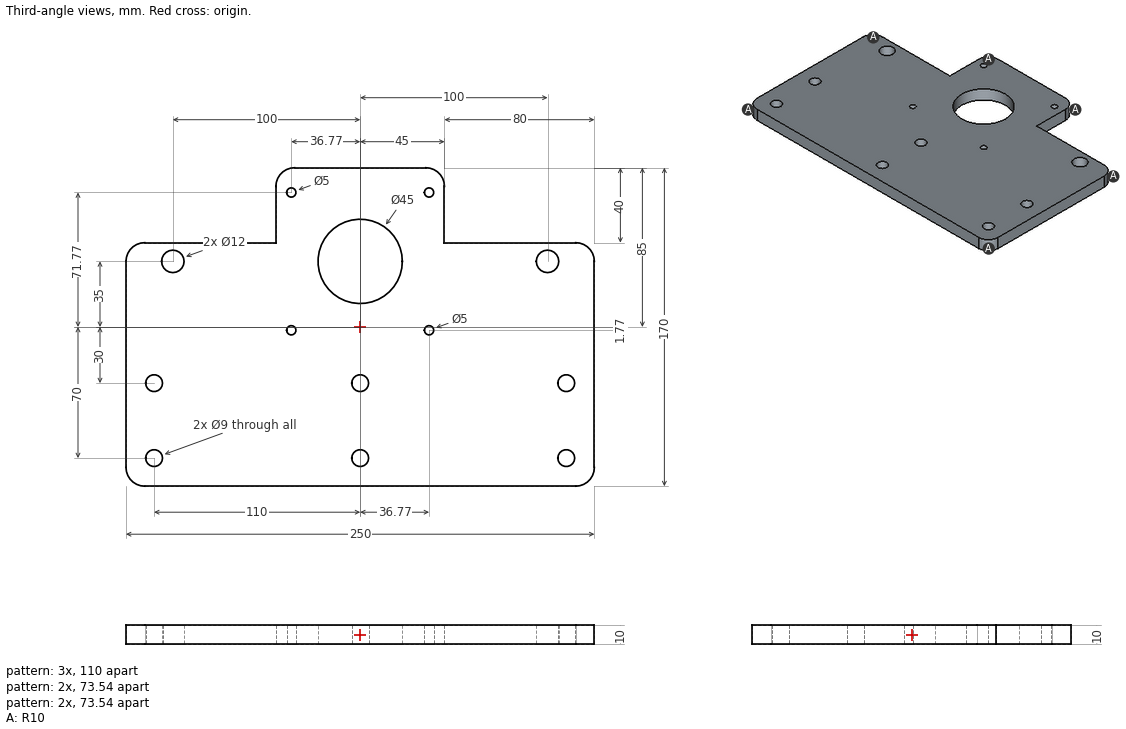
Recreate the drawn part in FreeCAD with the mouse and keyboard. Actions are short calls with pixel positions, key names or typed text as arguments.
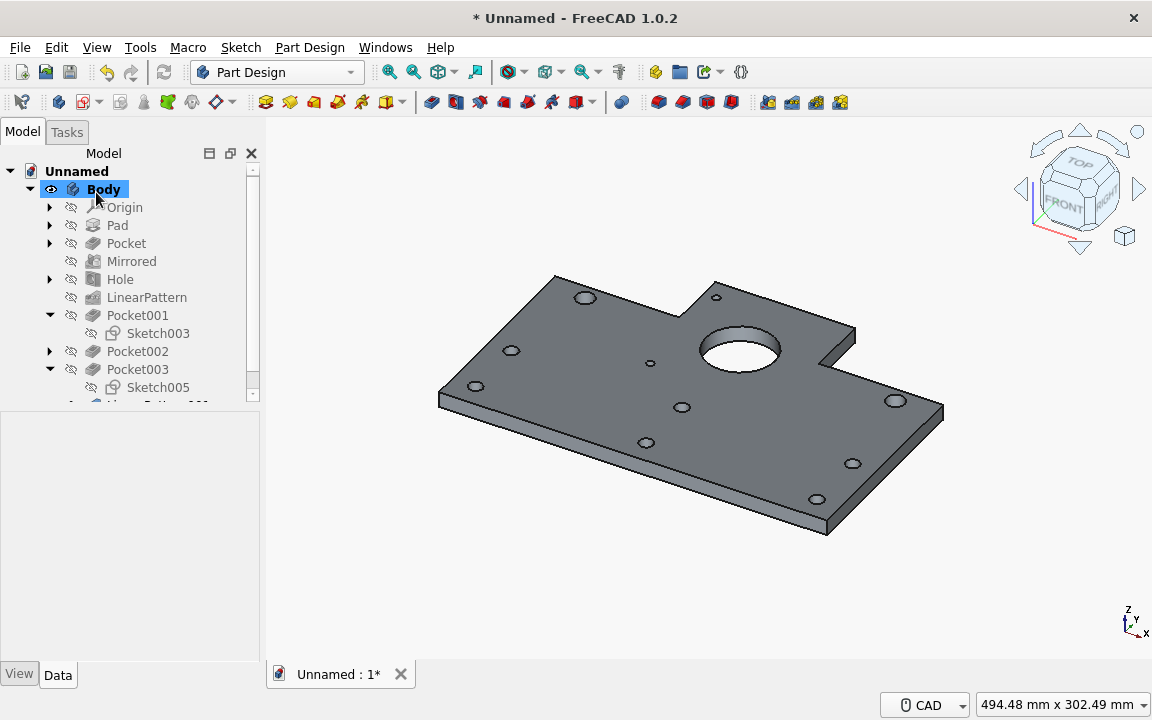
click(116, 369)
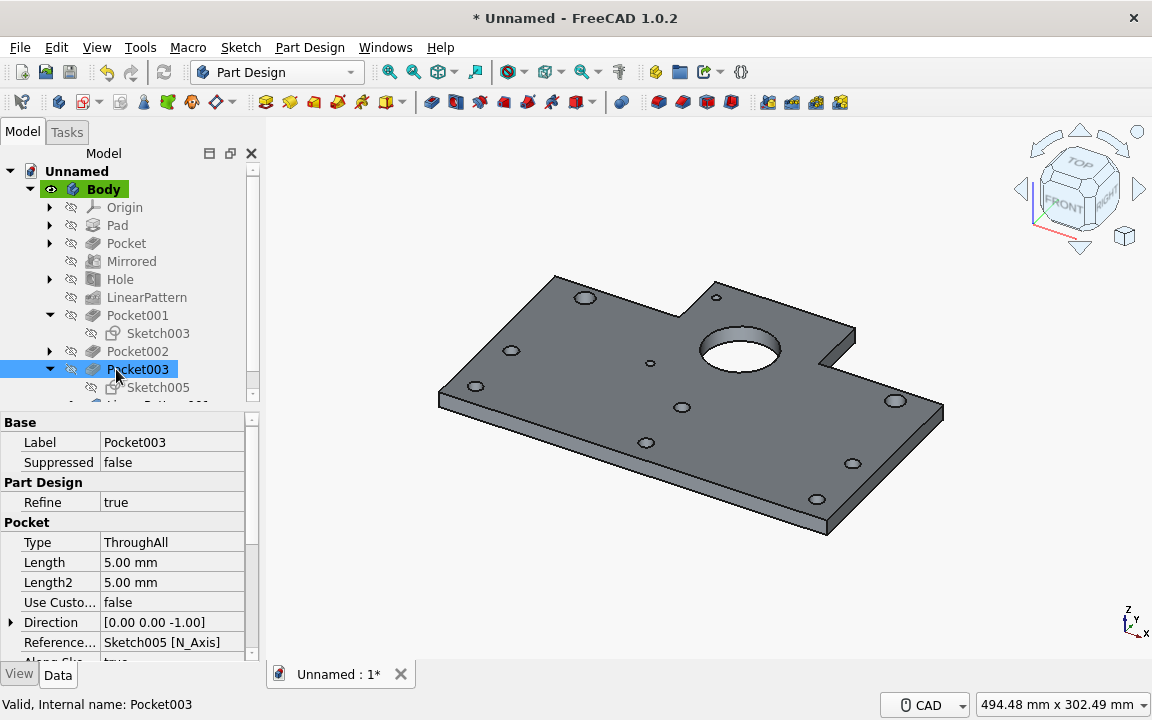
click(792, 102)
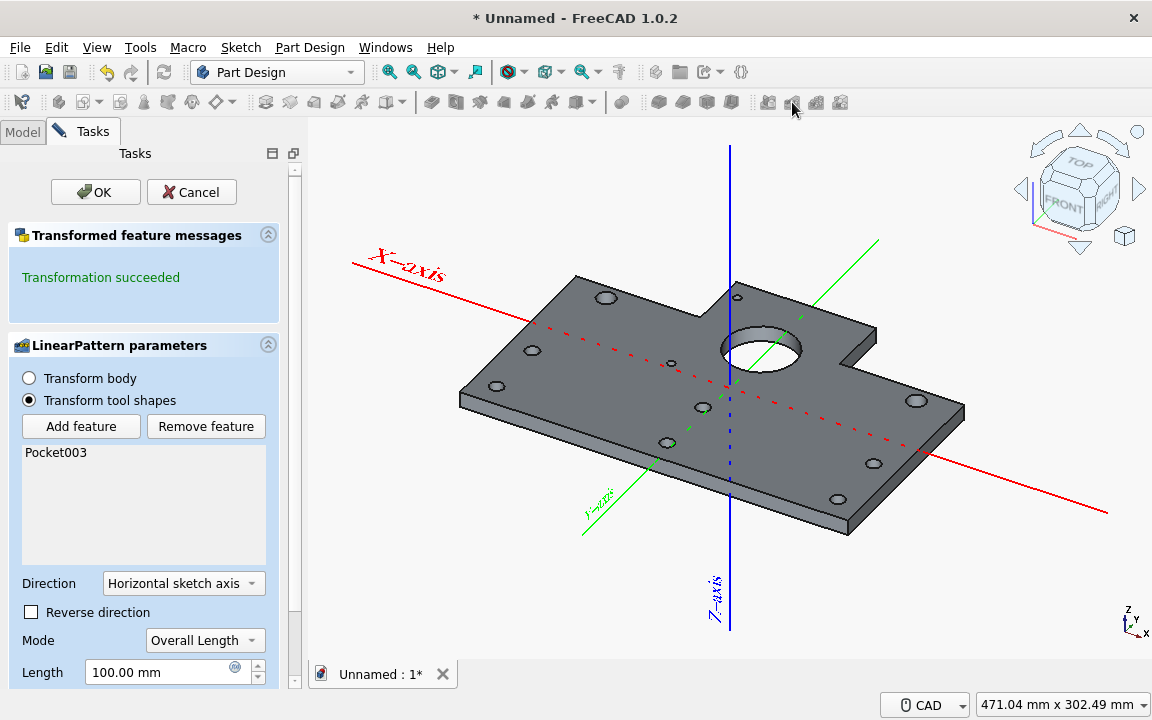
click(184, 584)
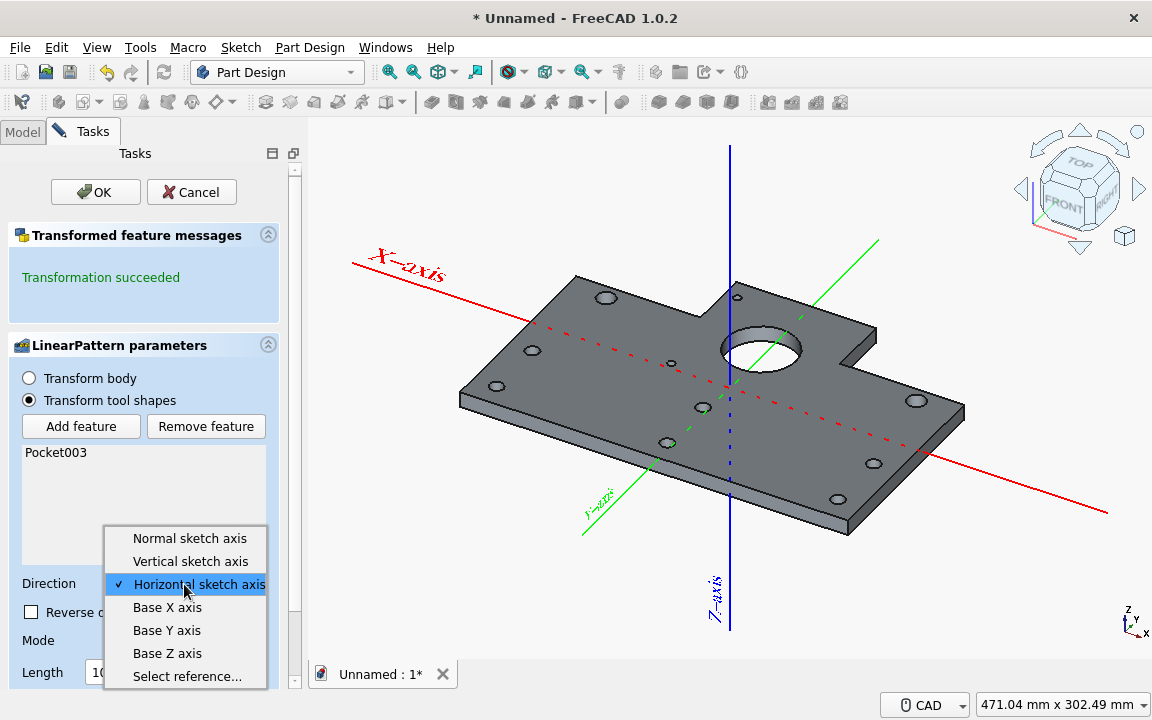
click(184, 608)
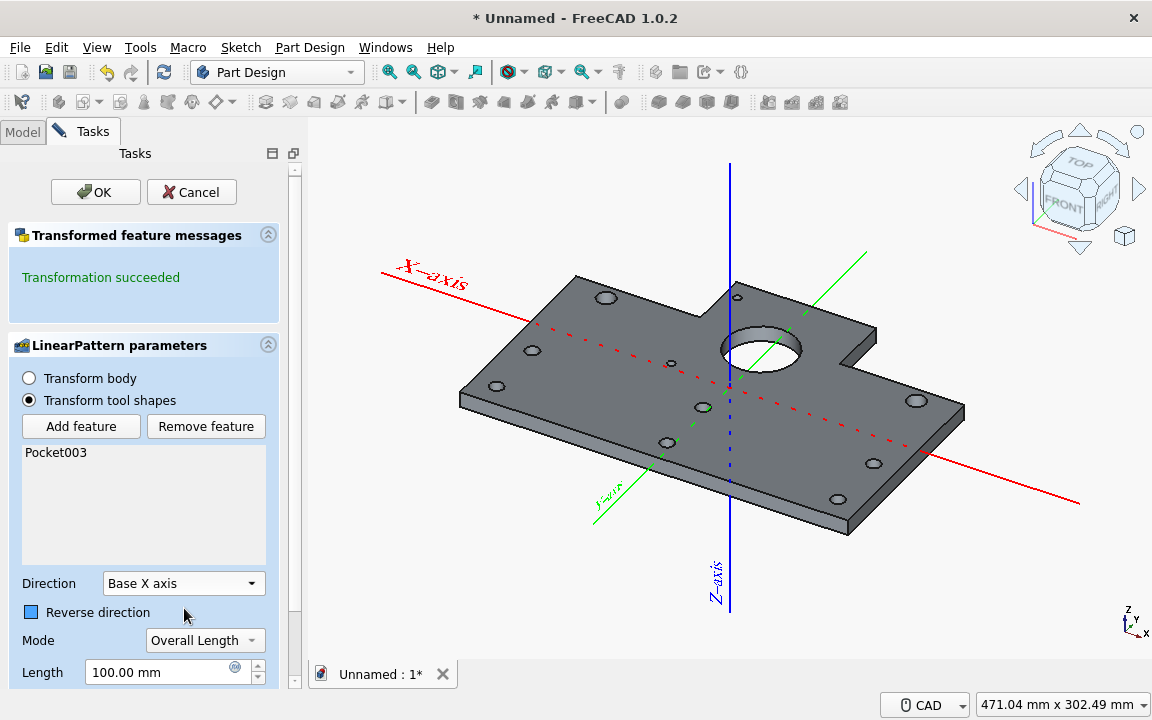
click(206, 640)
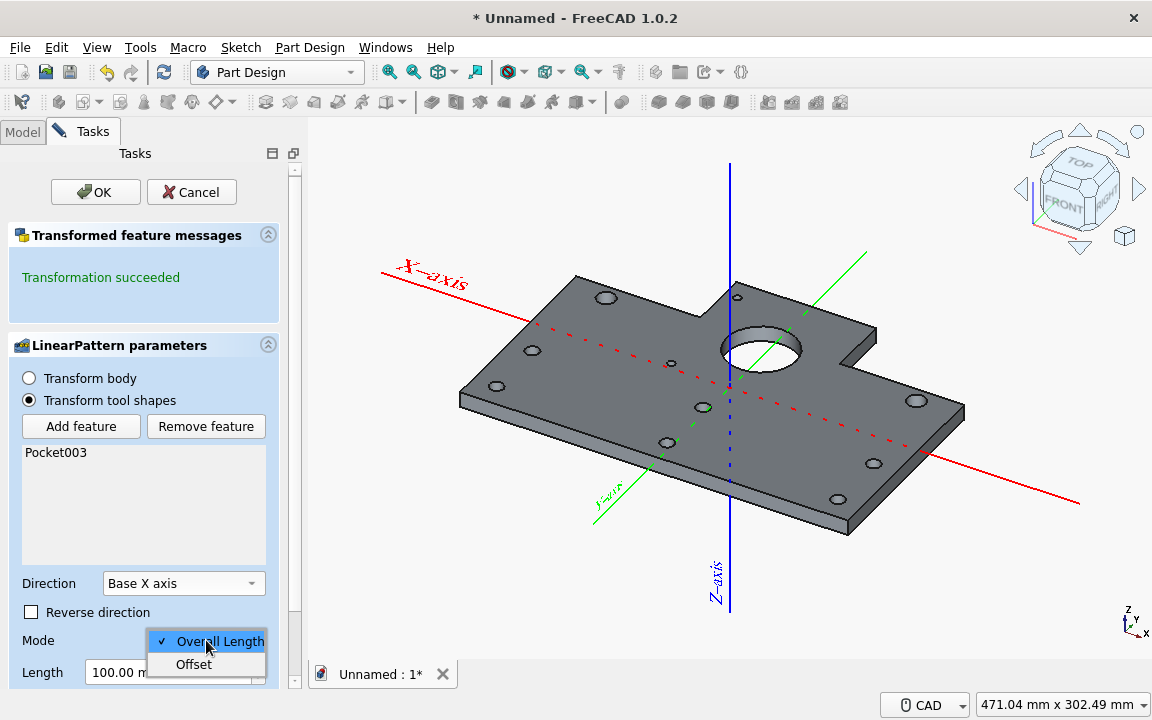
click(206, 664)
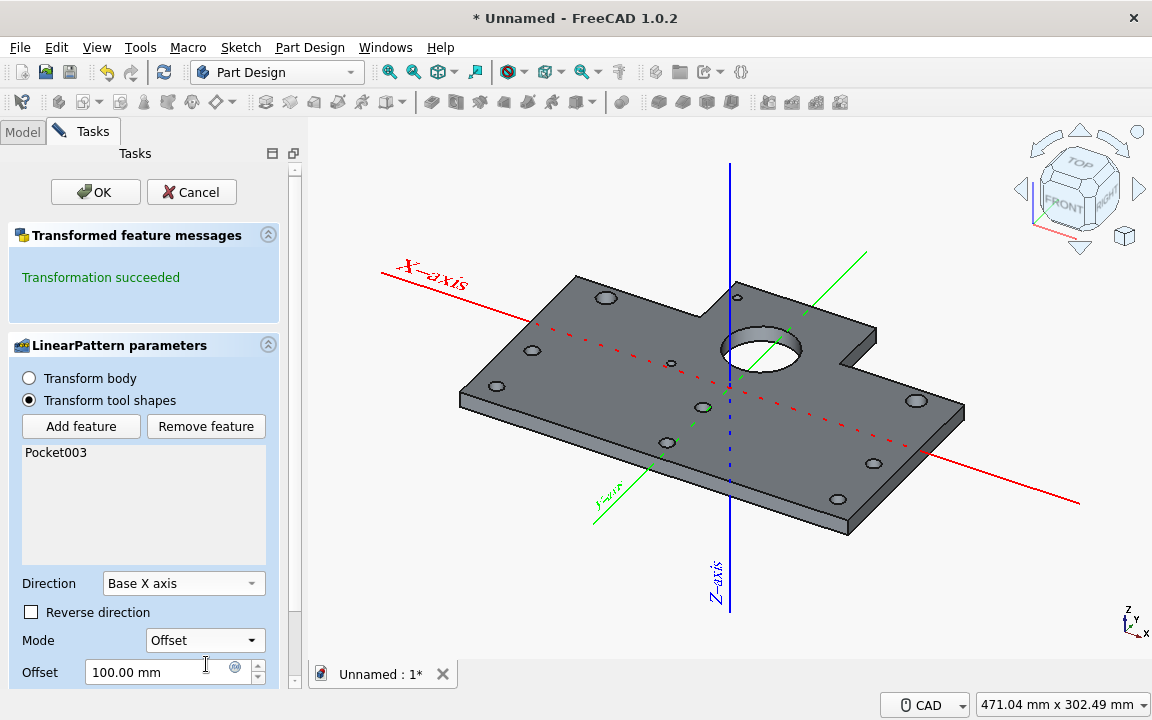
triple_click(168, 672)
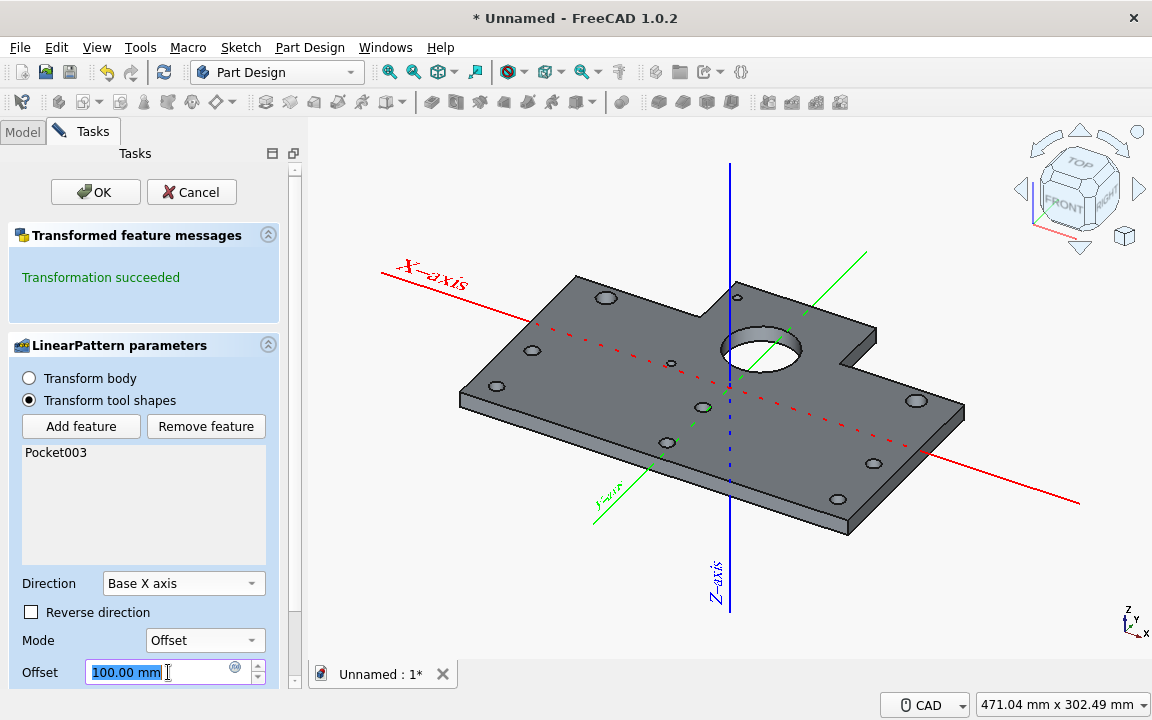
text(73.54)
key(Tab)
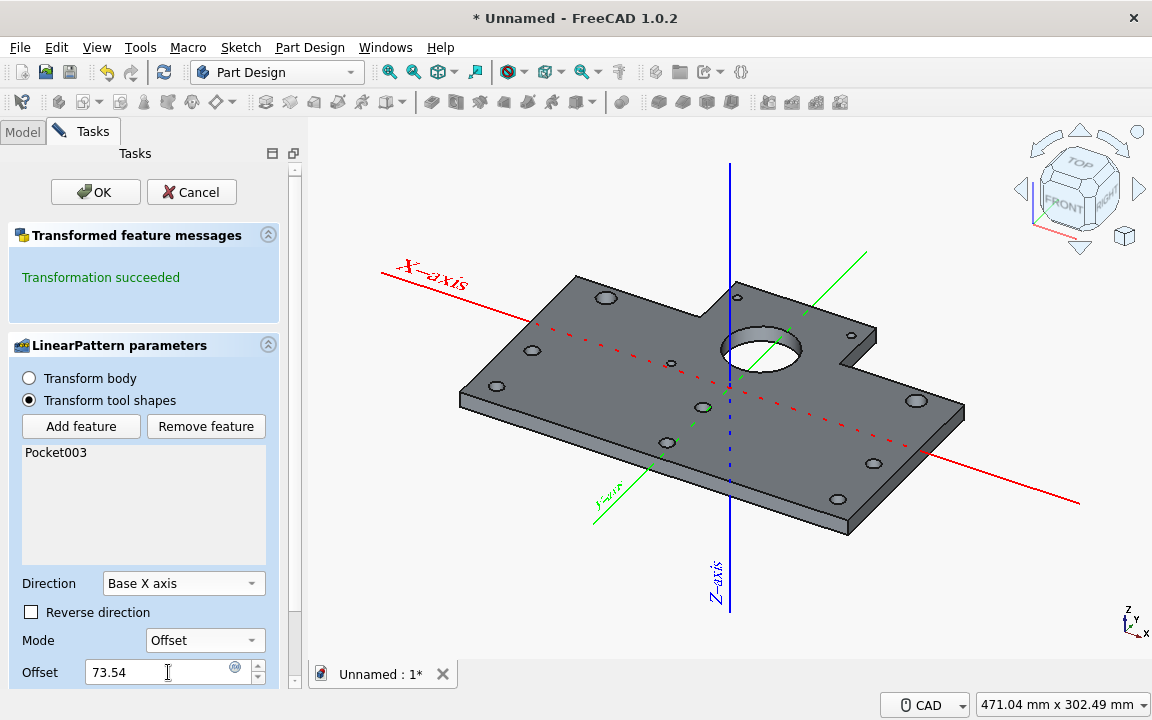
scroll(295, 426, down, 2)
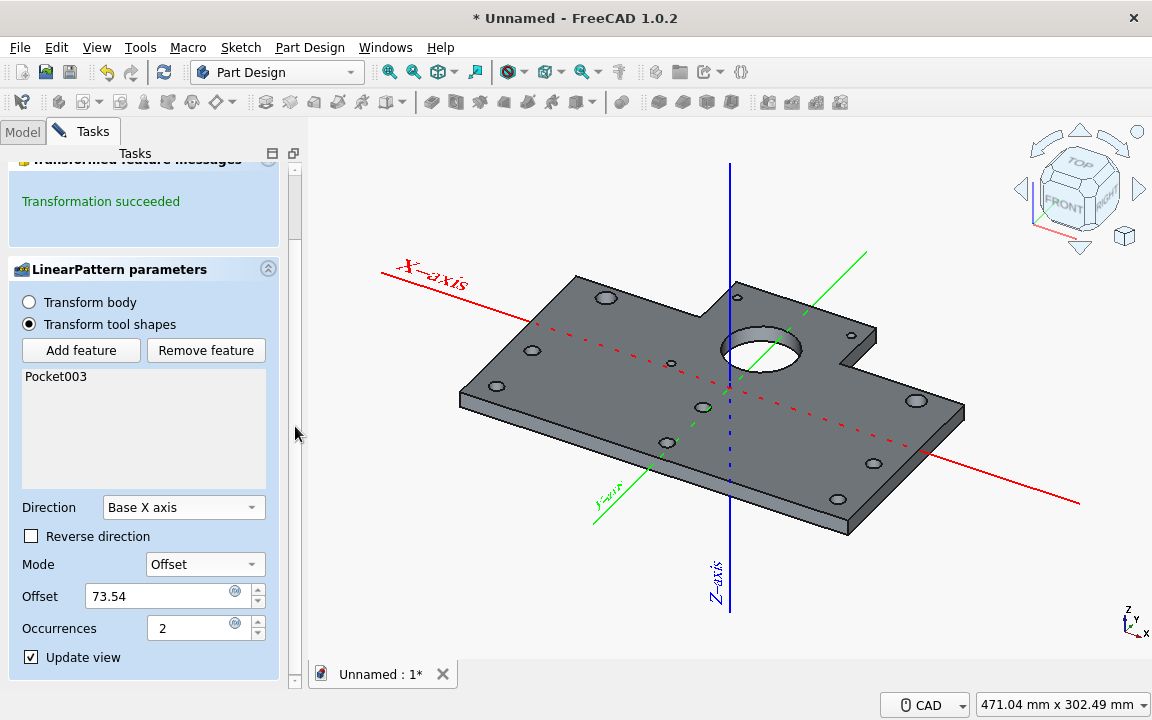
triple_click(198, 628)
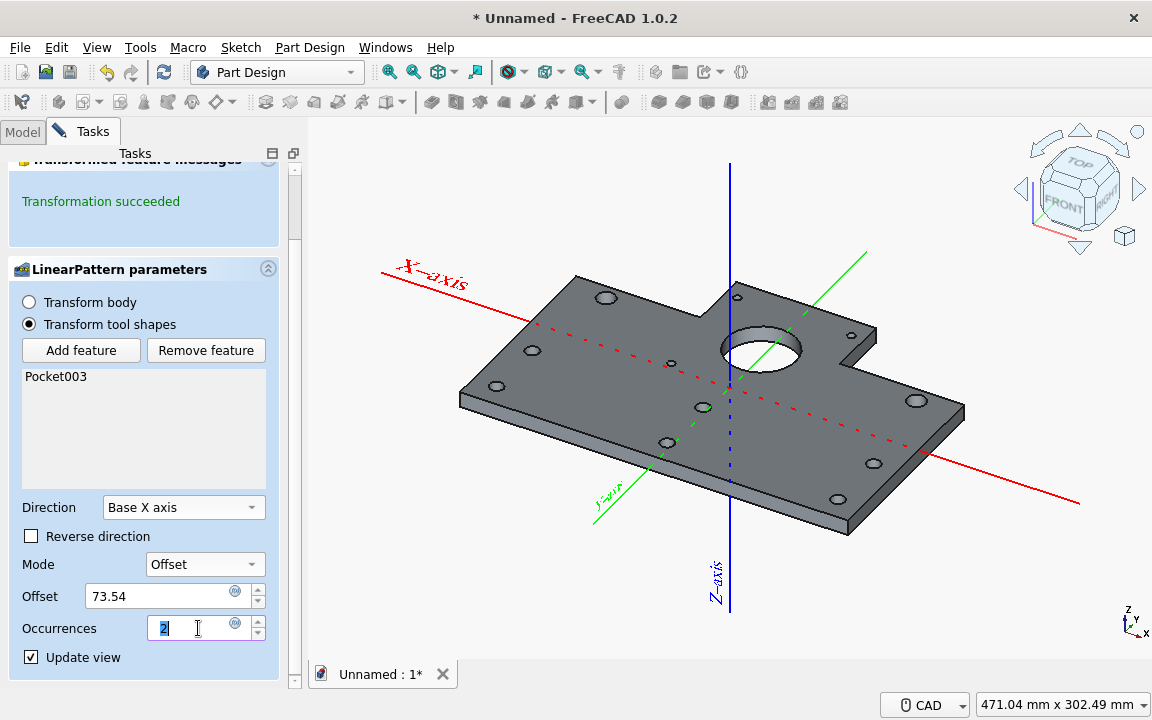
text(2)
key(Tab)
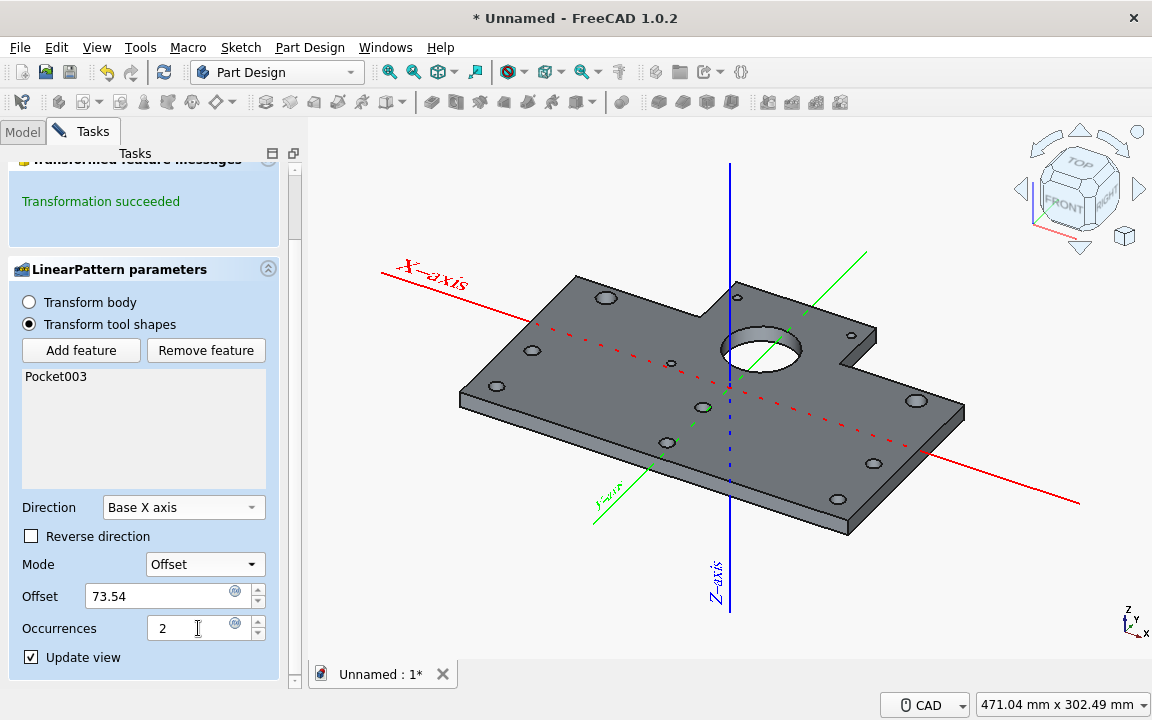
scroll(295, 426, up, 3)